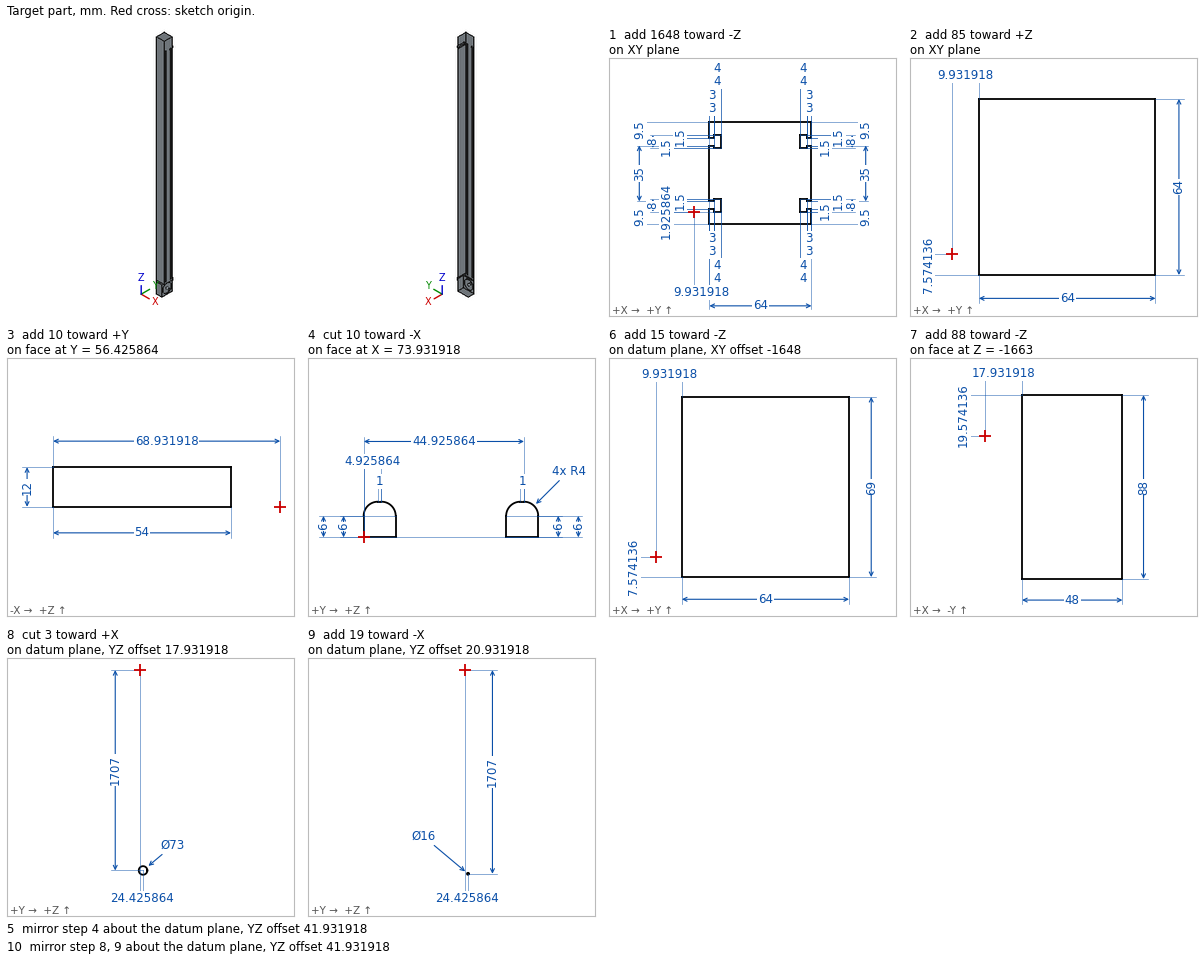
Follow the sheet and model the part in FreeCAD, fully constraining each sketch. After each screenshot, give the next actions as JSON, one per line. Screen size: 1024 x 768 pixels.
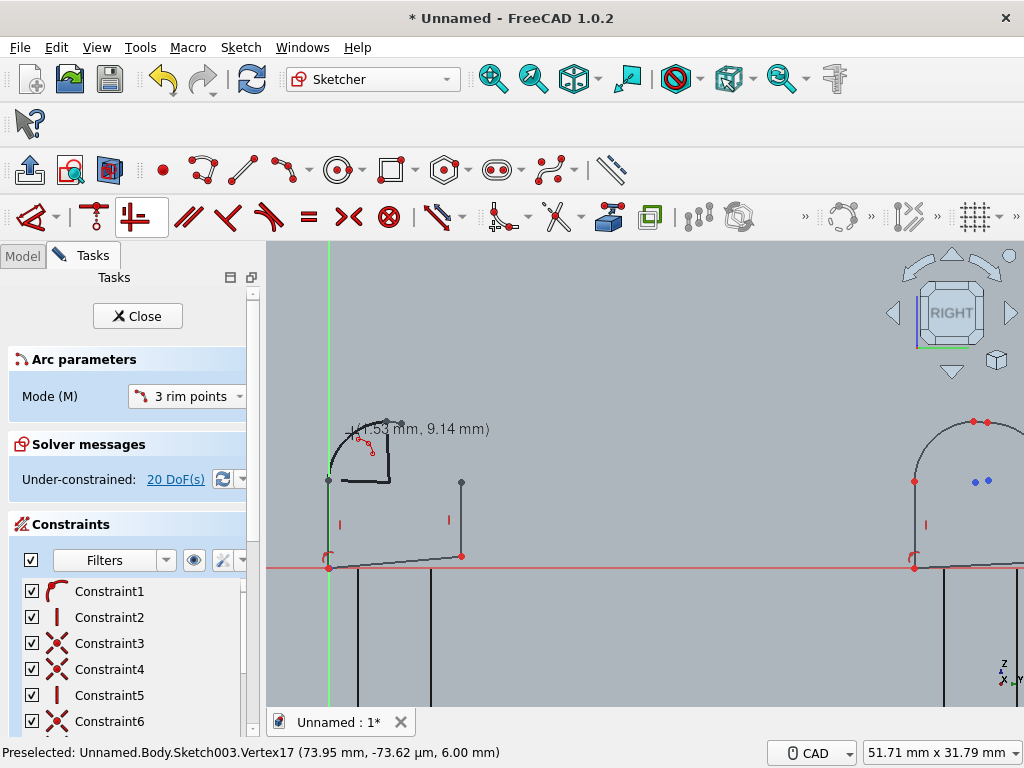
{"action": "left_click", "coordinate": [353, 433]}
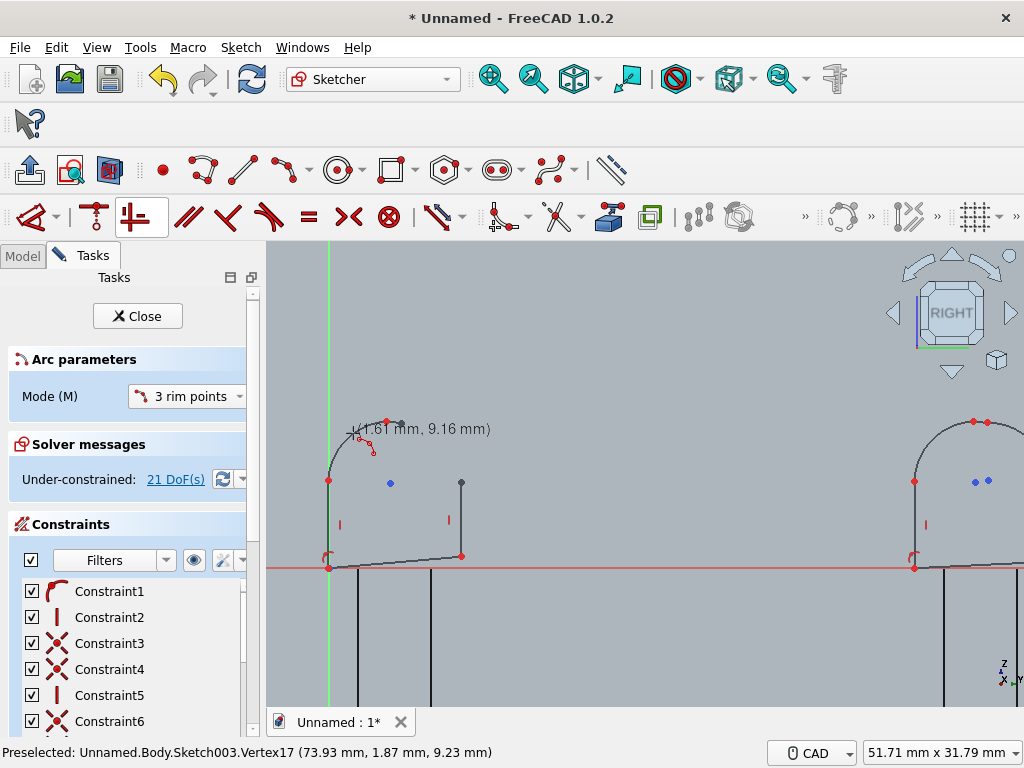
{"action": "left_click", "coordinate": [461, 482]}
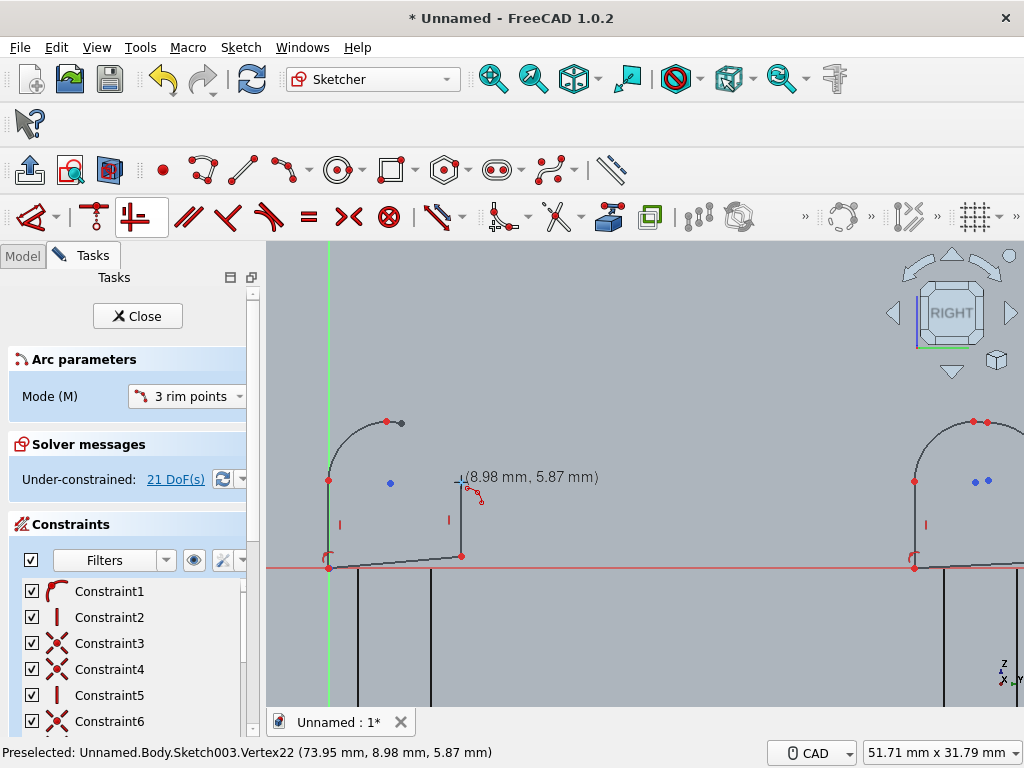
{"action": "scroll", "coordinate": [402, 422], "scroll_direction": "up", "scroll_amount": 4}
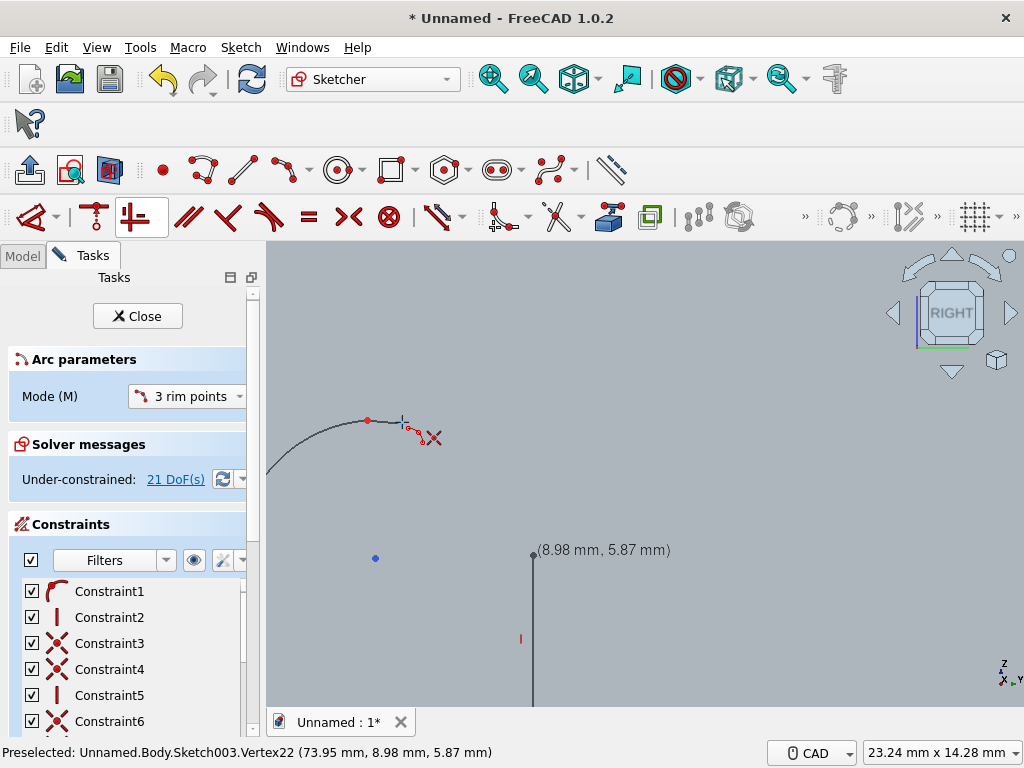
{"action": "left_click", "coordinate": [402, 424]}
{"action": "left_click", "coordinate": [493, 459]}
{"action": "key", "text": "Escape"}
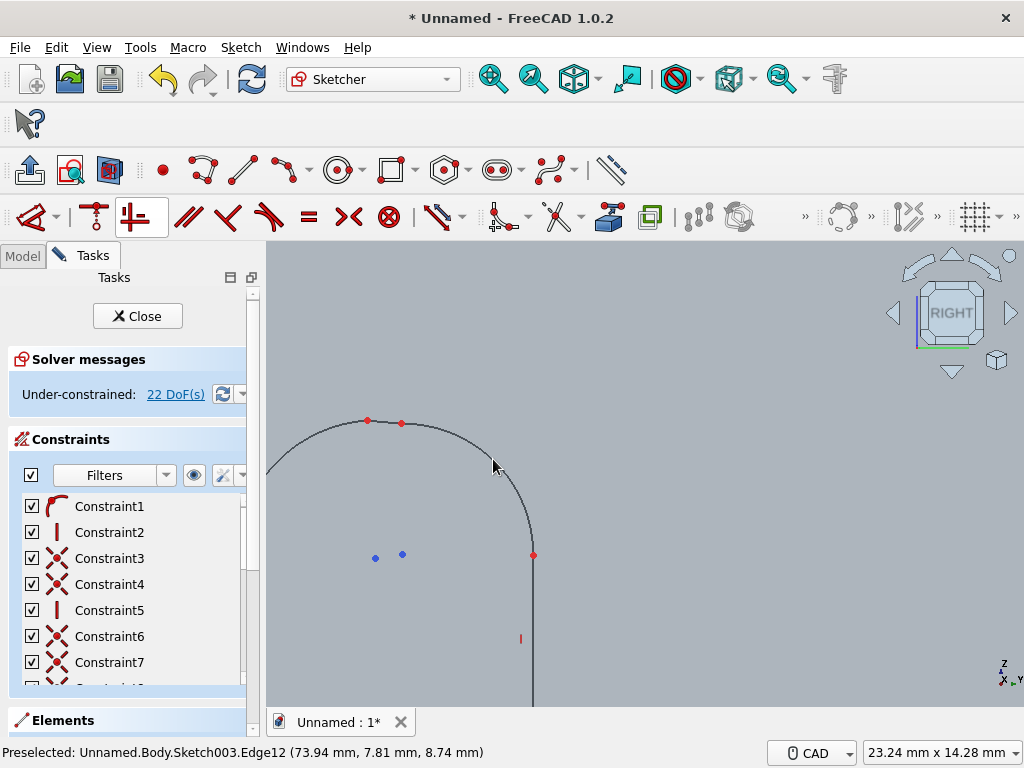
{"action": "scroll", "coordinate": [426, 438], "scroll_direction": "down", "scroll_amount": 7}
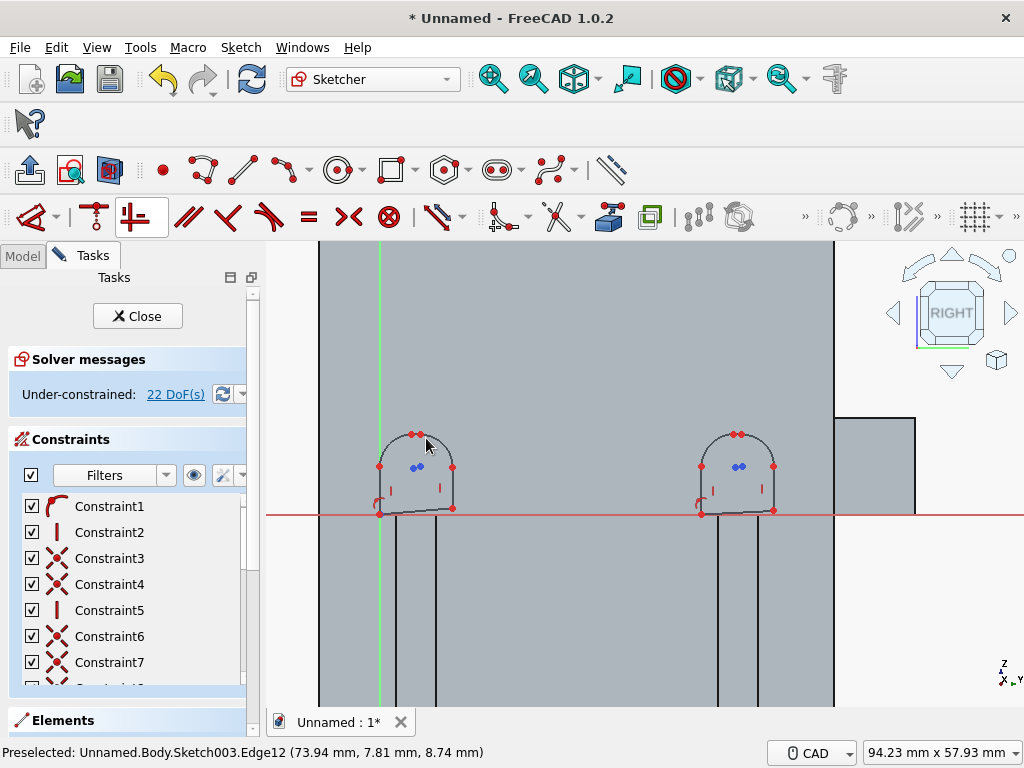
{"action": "scroll", "coordinate": [739, 435], "scroll_direction": "up", "scroll_amount": 9}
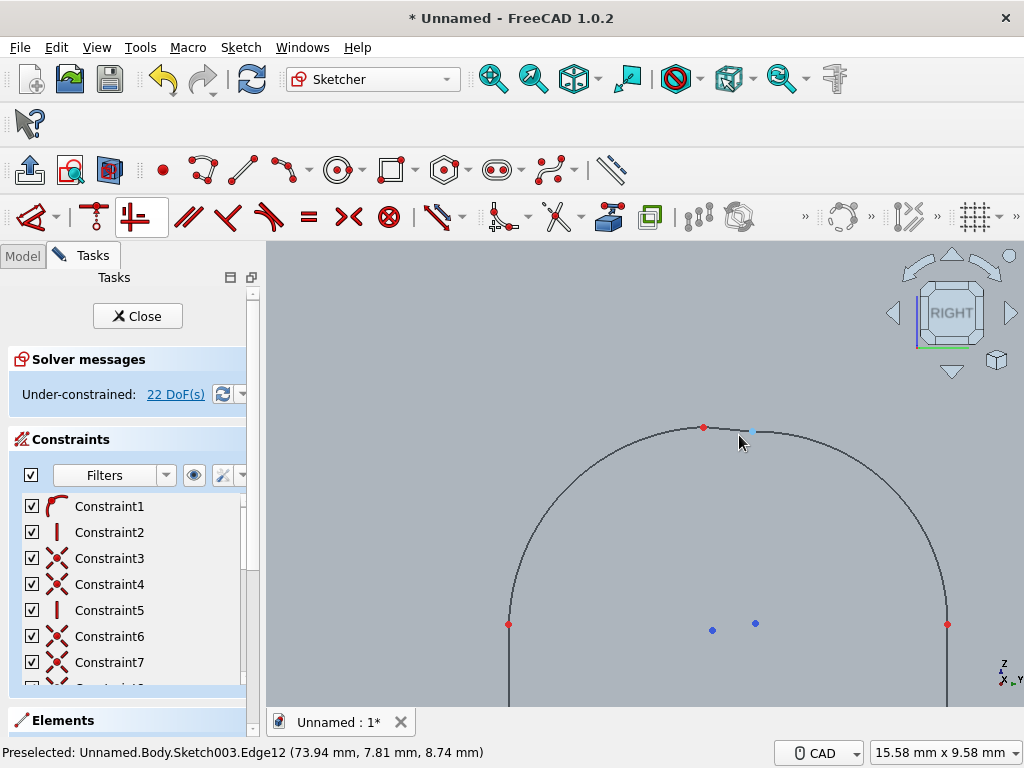
{"action": "left_click", "coordinate": [738, 430]}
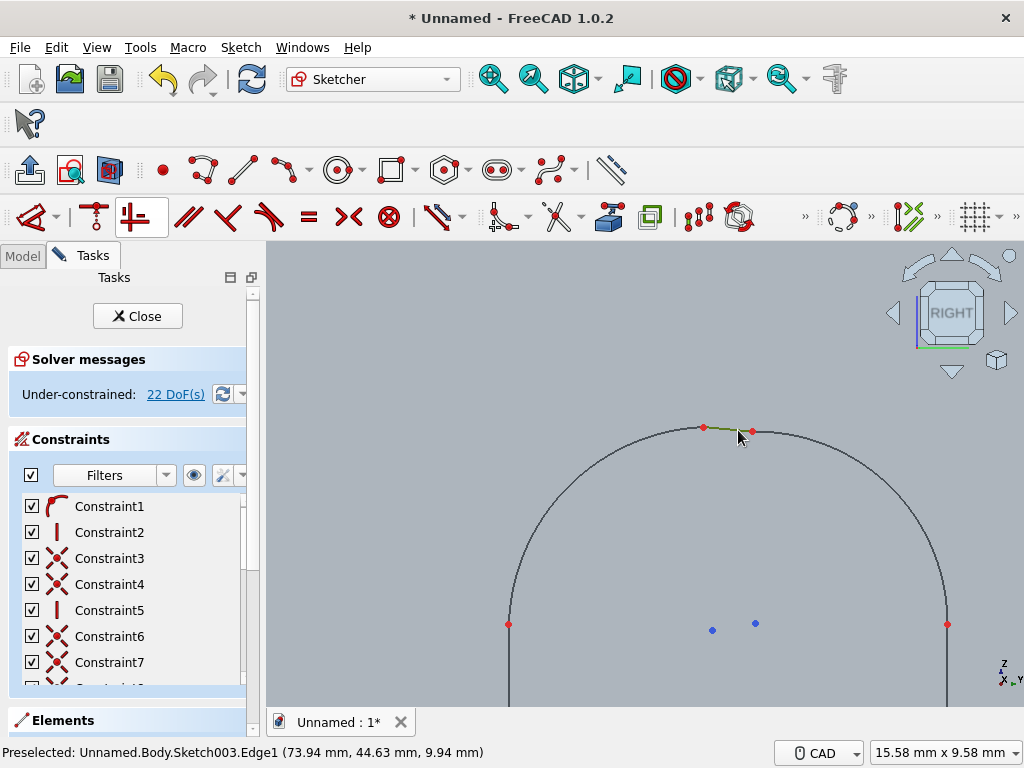
{"action": "scroll", "coordinate": [739, 435], "scroll_direction": "down", "scroll_amount": 9}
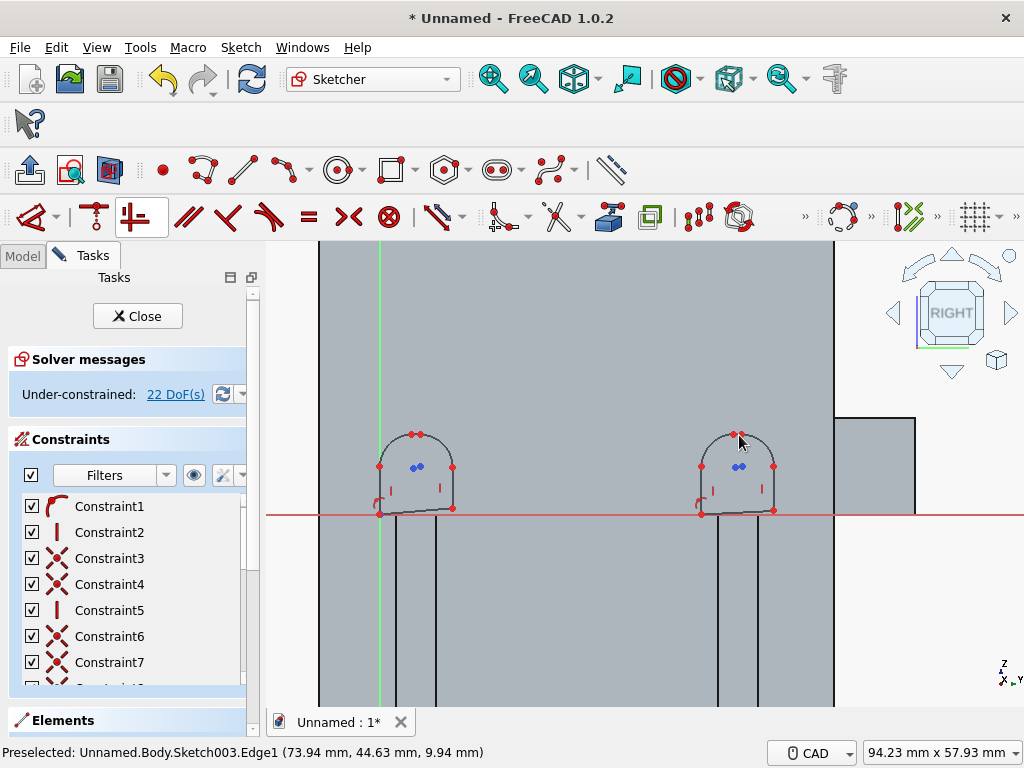
{"action": "left_click", "coordinate": [719, 438]}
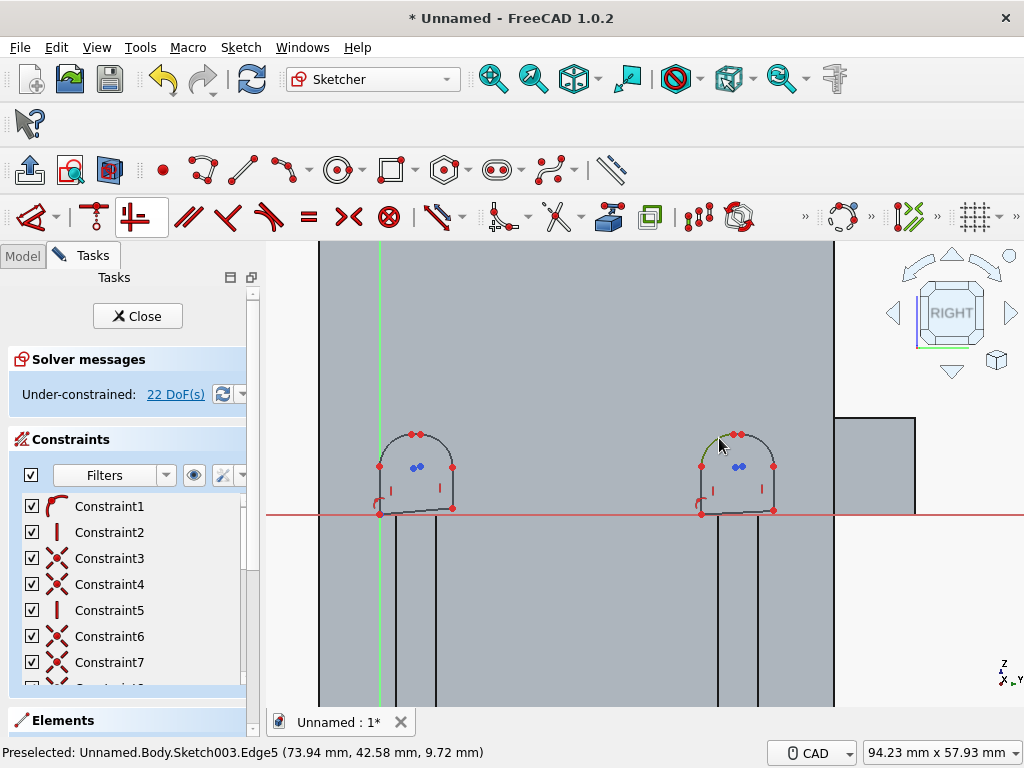
{"action": "left_click", "coordinate": [270, 218]}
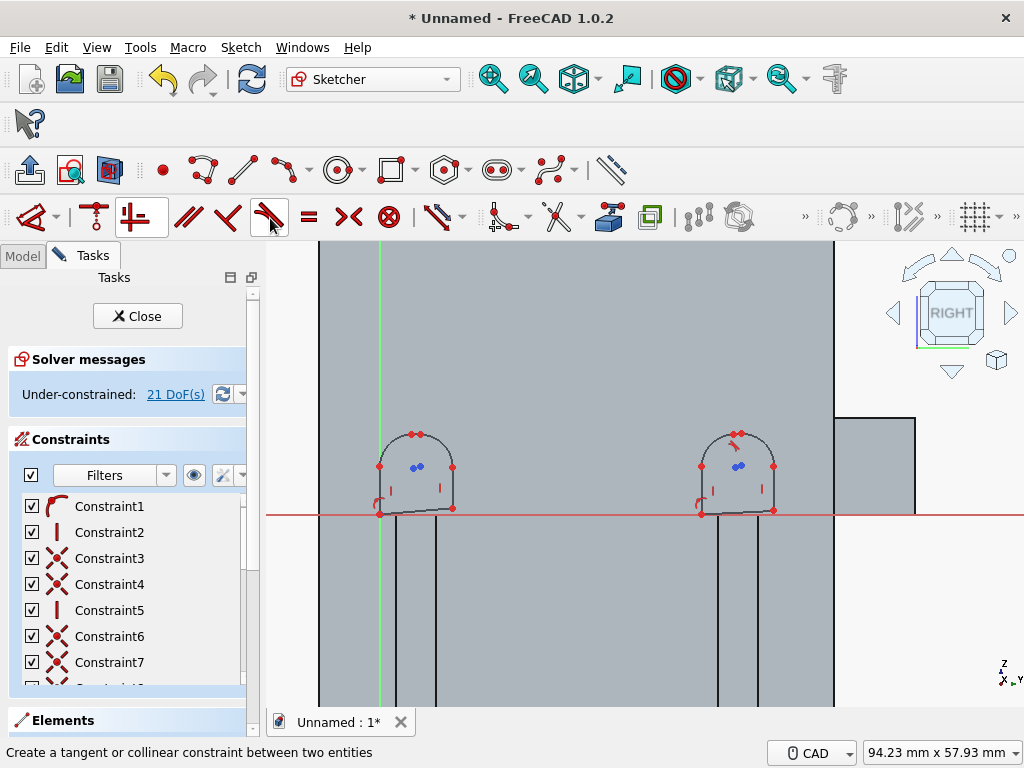
{"action": "scroll", "coordinate": [738, 434], "scroll_direction": "up", "scroll_amount": 7}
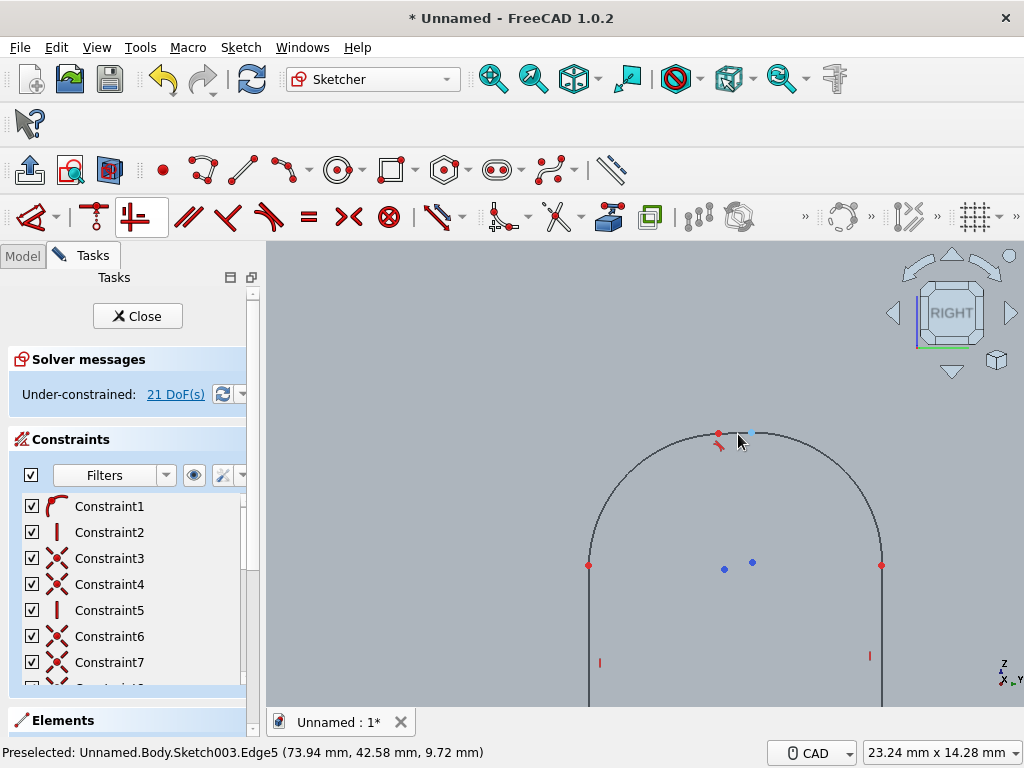
{"action": "left_click", "coordinate": [735, 433]}